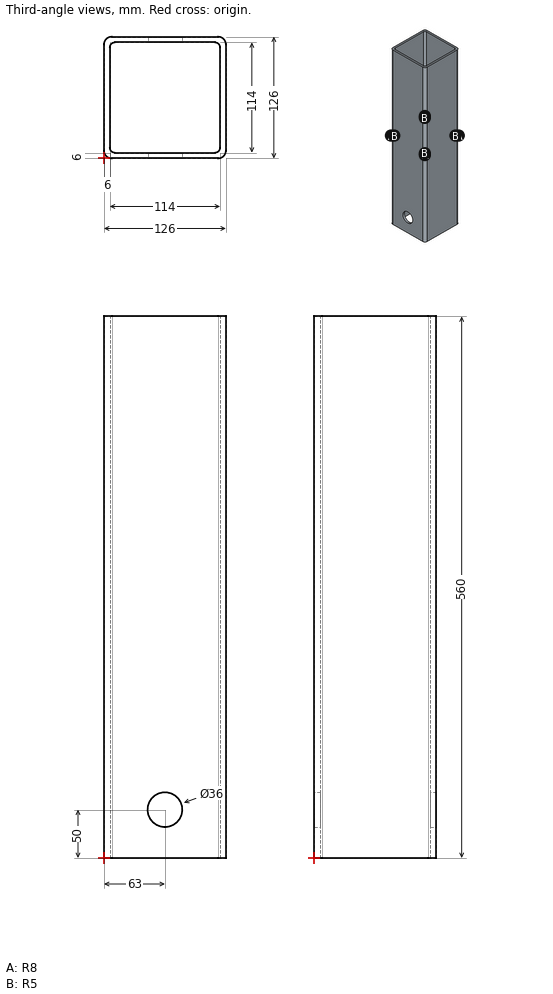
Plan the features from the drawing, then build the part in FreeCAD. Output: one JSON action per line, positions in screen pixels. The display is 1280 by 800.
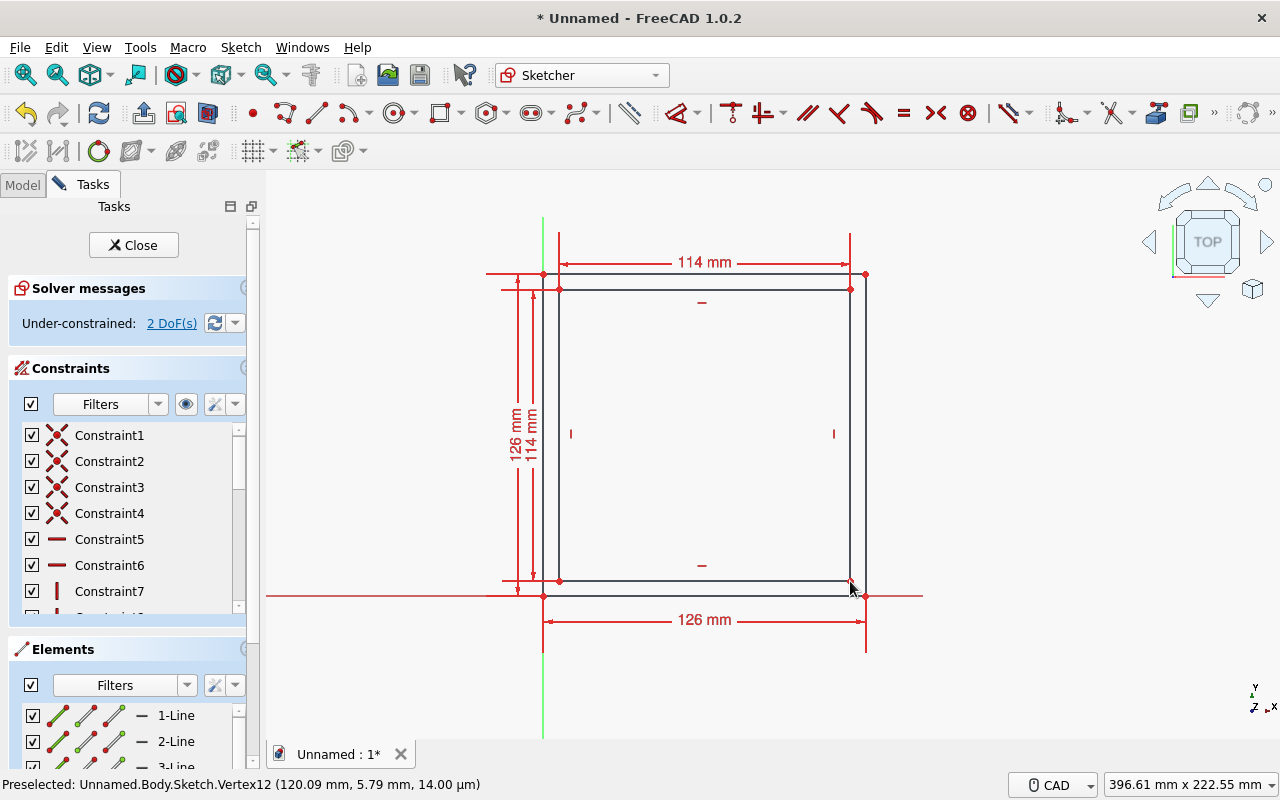
{"action": "scroll", "coordinate": [559, 290], "scroll_direction": "up", "scroll_amount": 5}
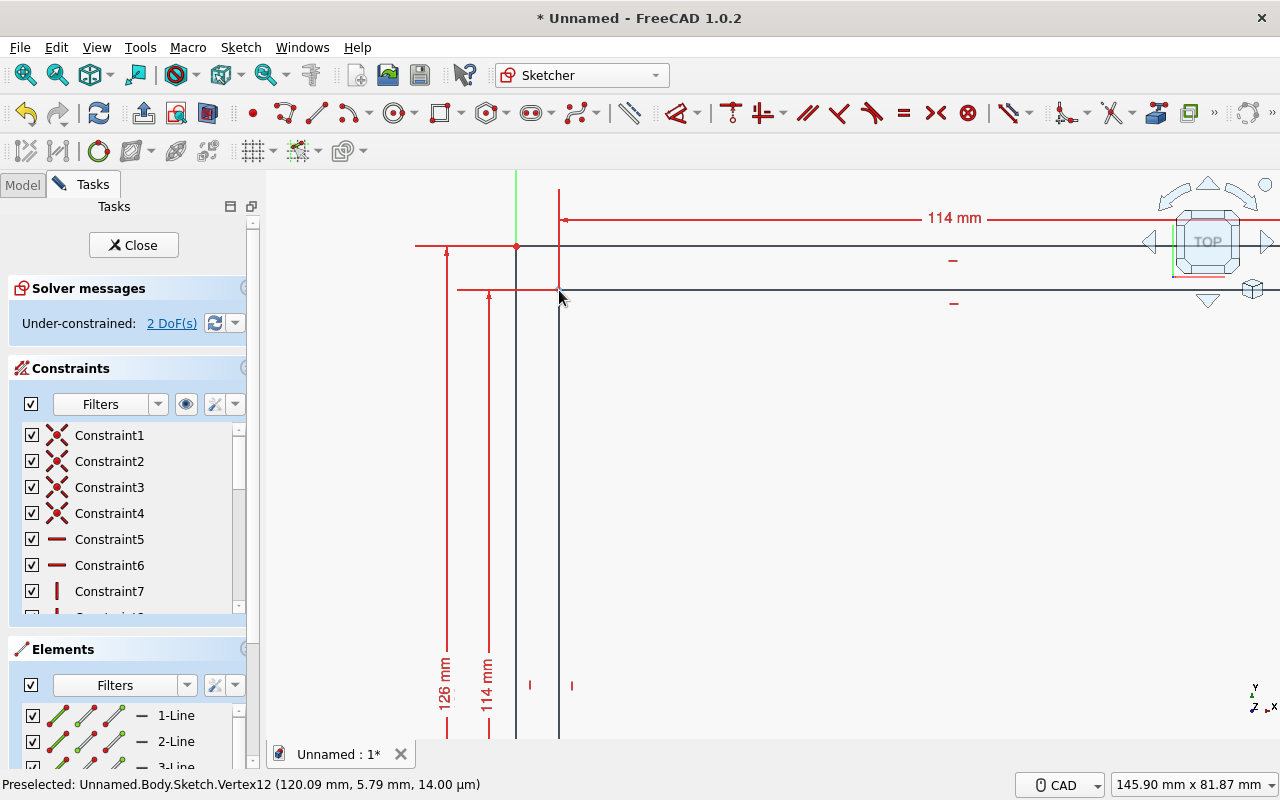
{"action": "left_click", "coordinate": [559, 290]}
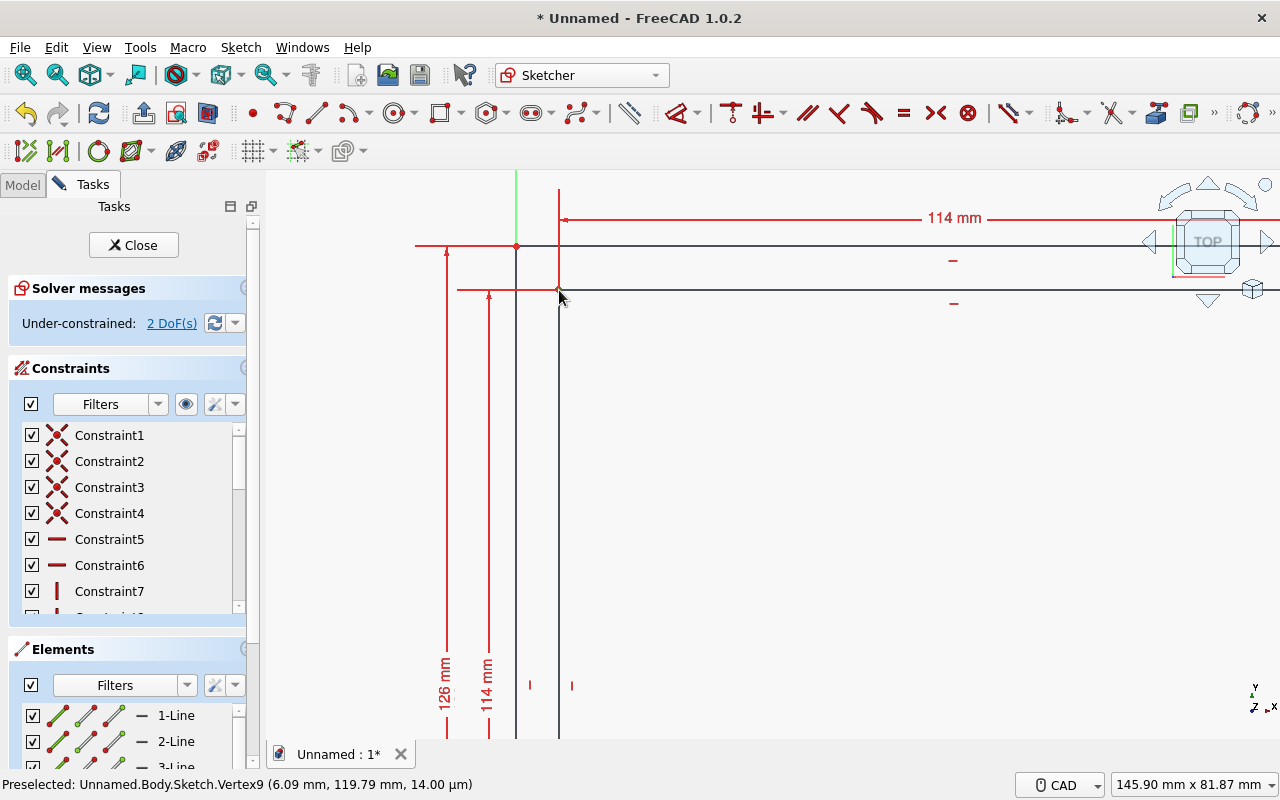
{"action": "left_click", "coordinate": [700, 114]}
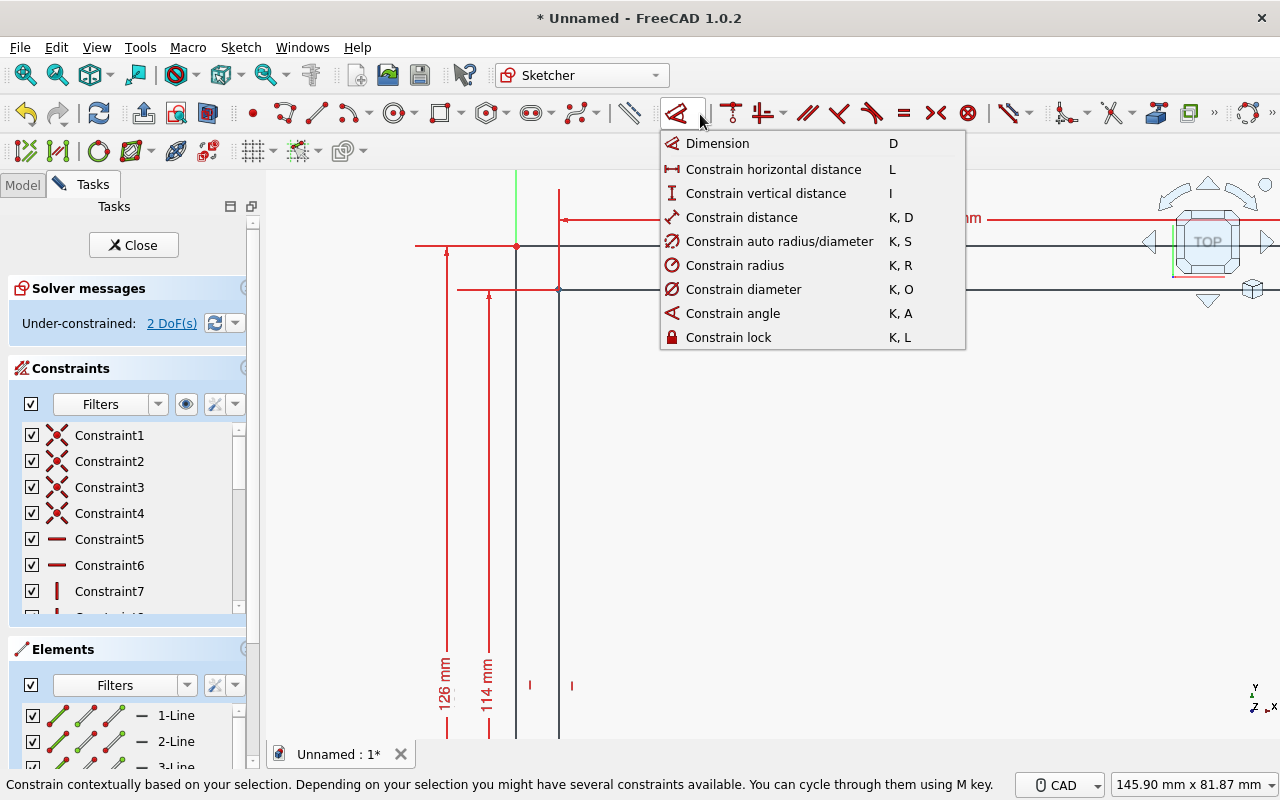
{"action": "left_click", "coordinate": [813, 169]}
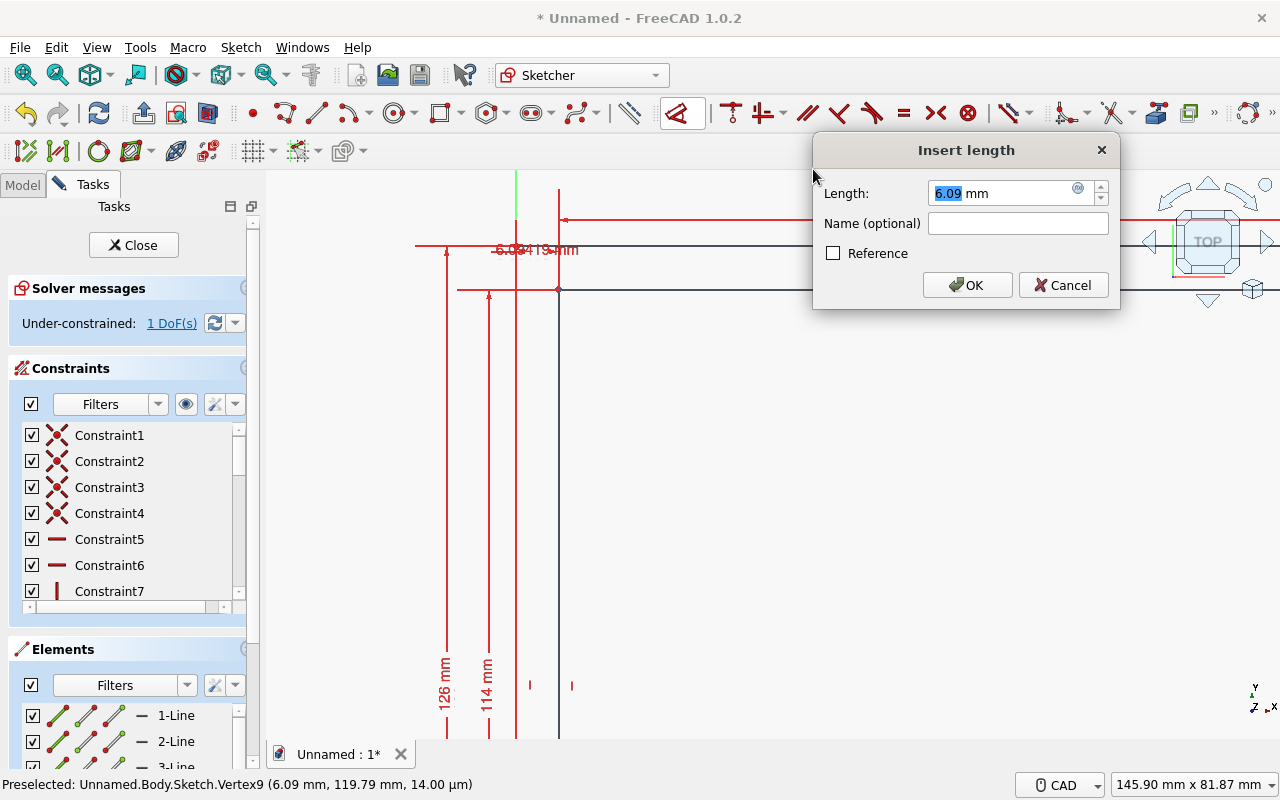
{"action": "type", "text": "6"}
{"action": "key", "text": "Return"}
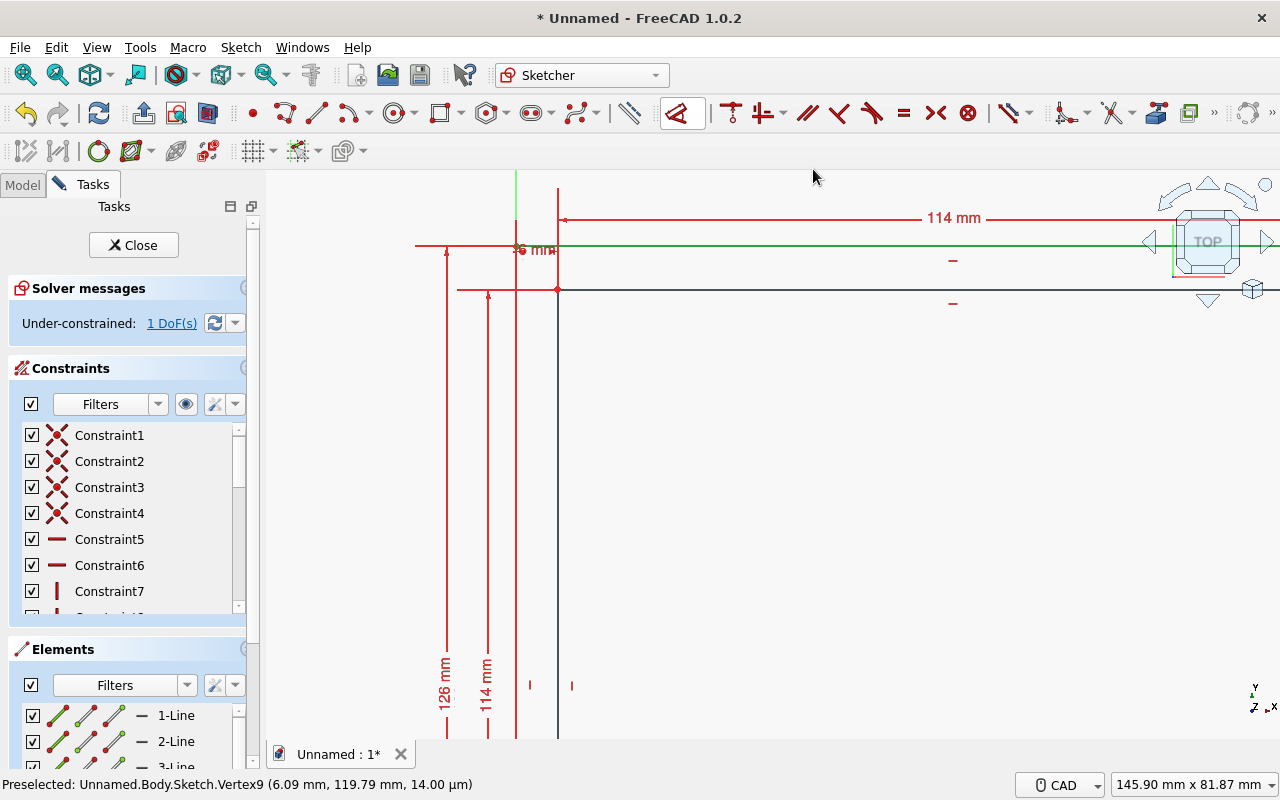
{"action": "scroll", "coordinate": [501, 267], "scroll_direction": "down", "scroll_amount": 4}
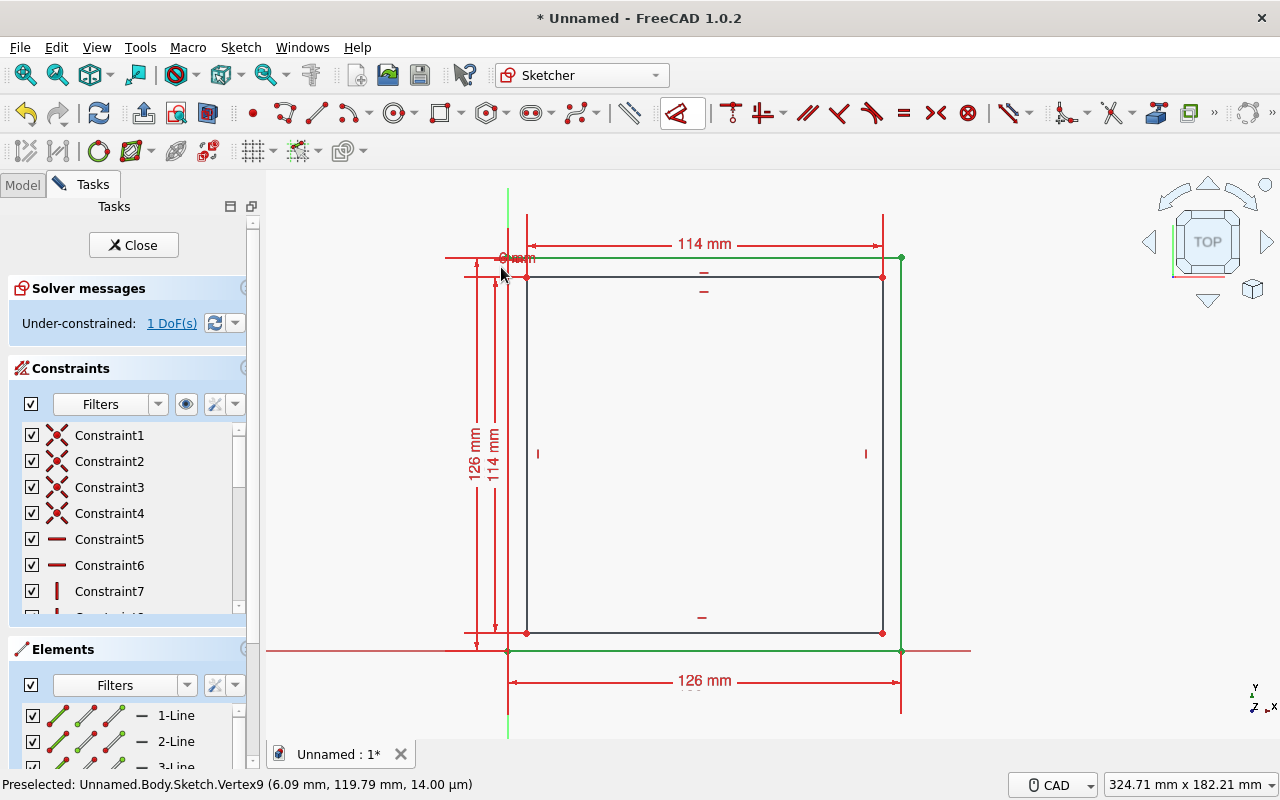
{"action": "scroll", "coordinate": [527, 633], "scroll_direction": "up", "scroll_amount": 4}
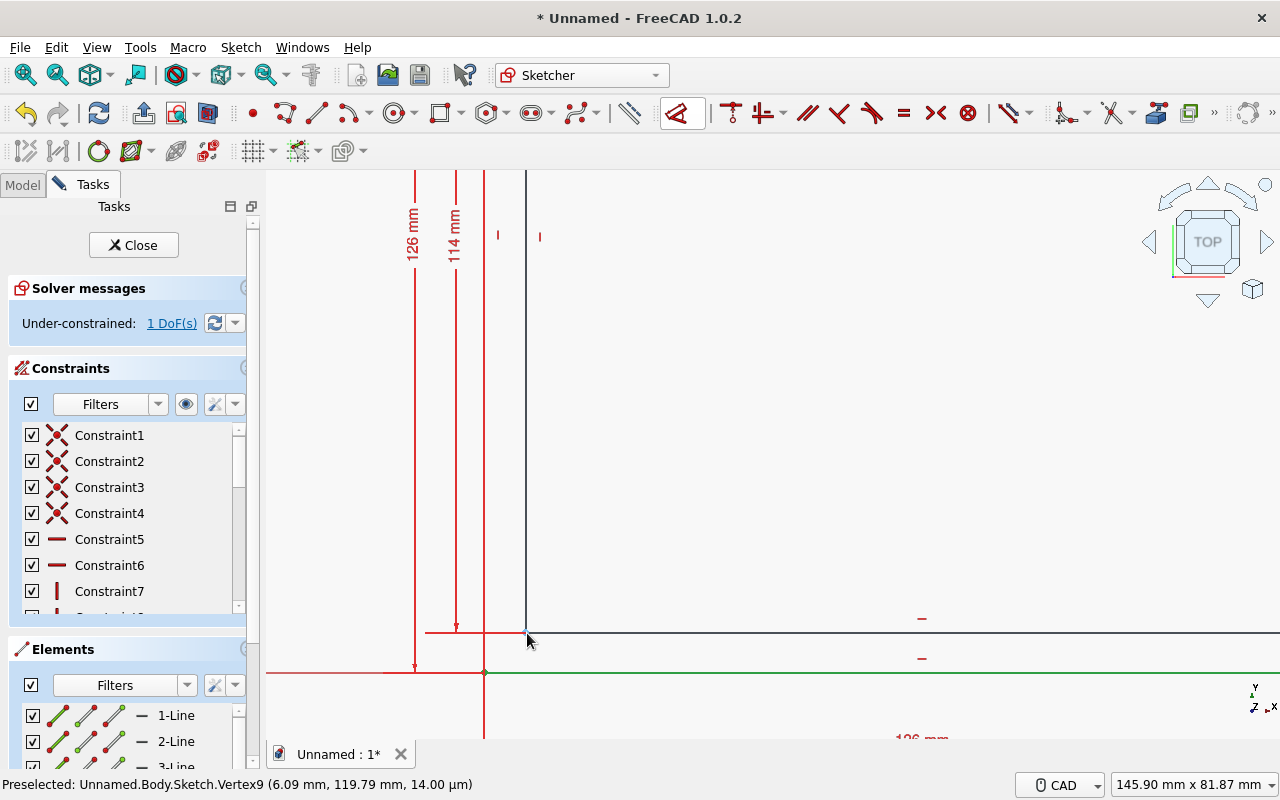
{"action": "left_click", "coordinate": [526, 633]}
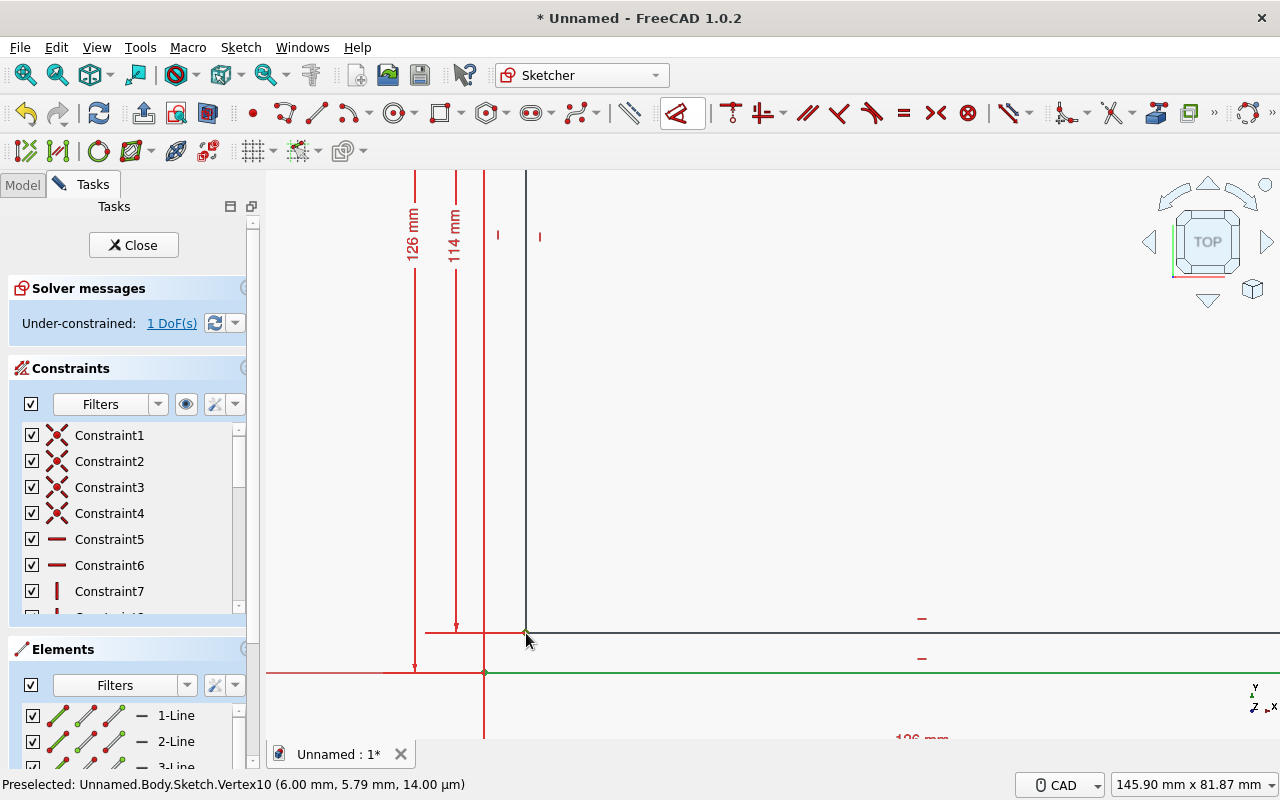
{"action": "left_click", "coordinate": [700, 114]}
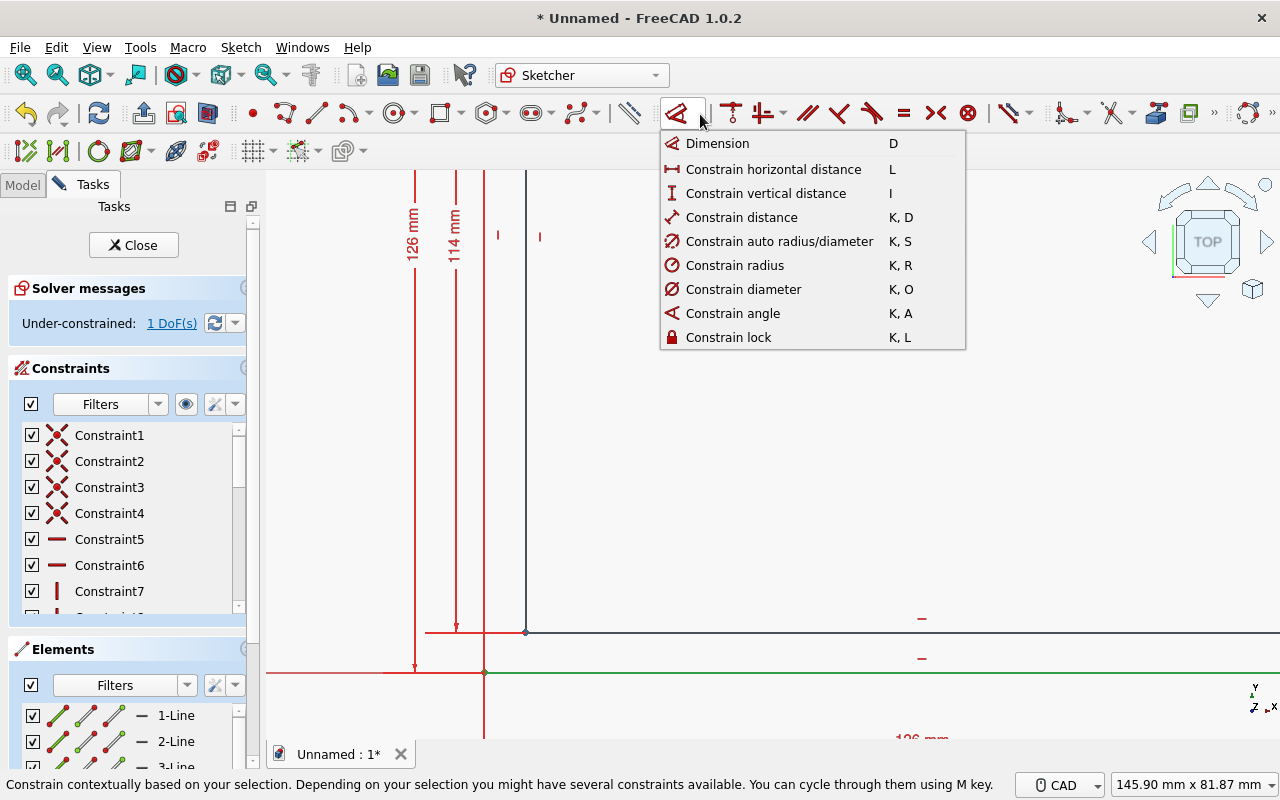
{"action": "left_click", "coordinate": [813, 193]}